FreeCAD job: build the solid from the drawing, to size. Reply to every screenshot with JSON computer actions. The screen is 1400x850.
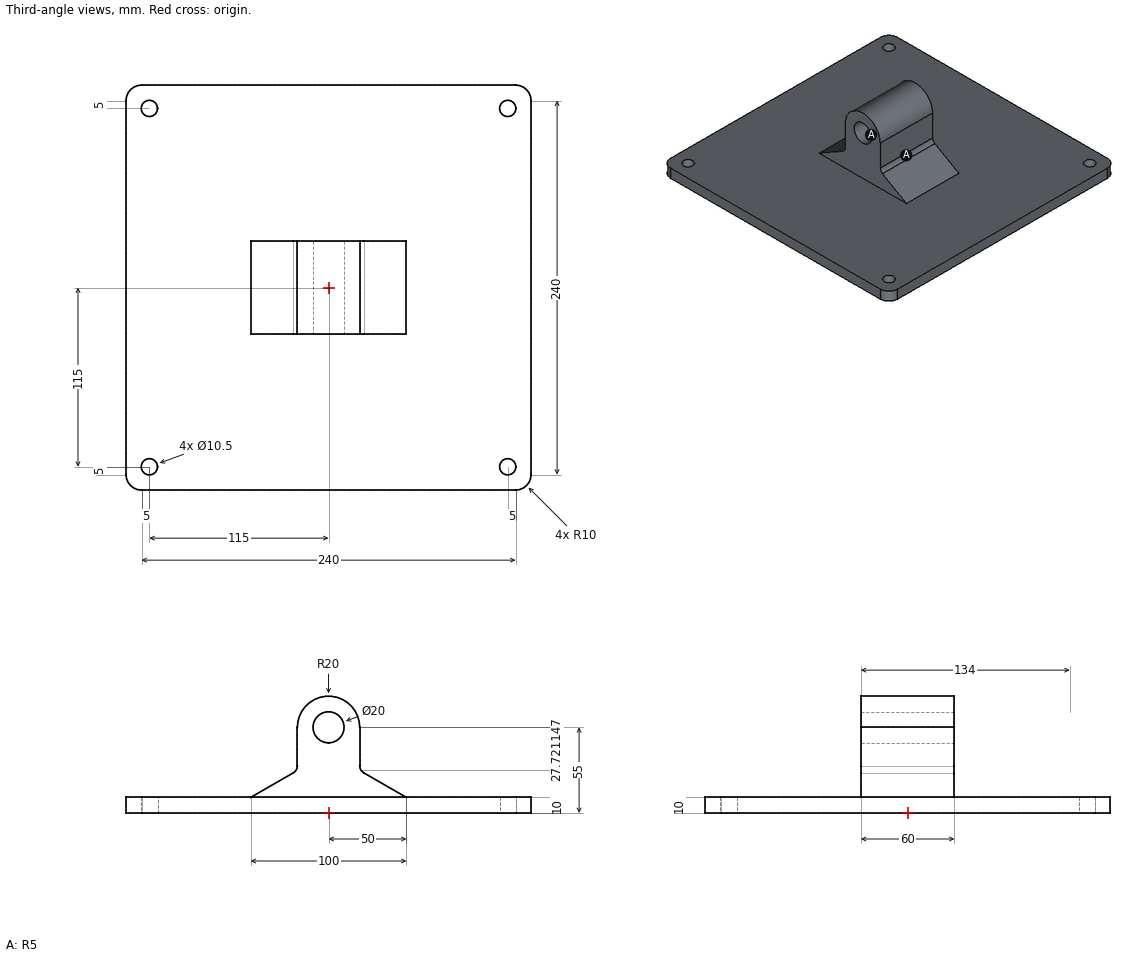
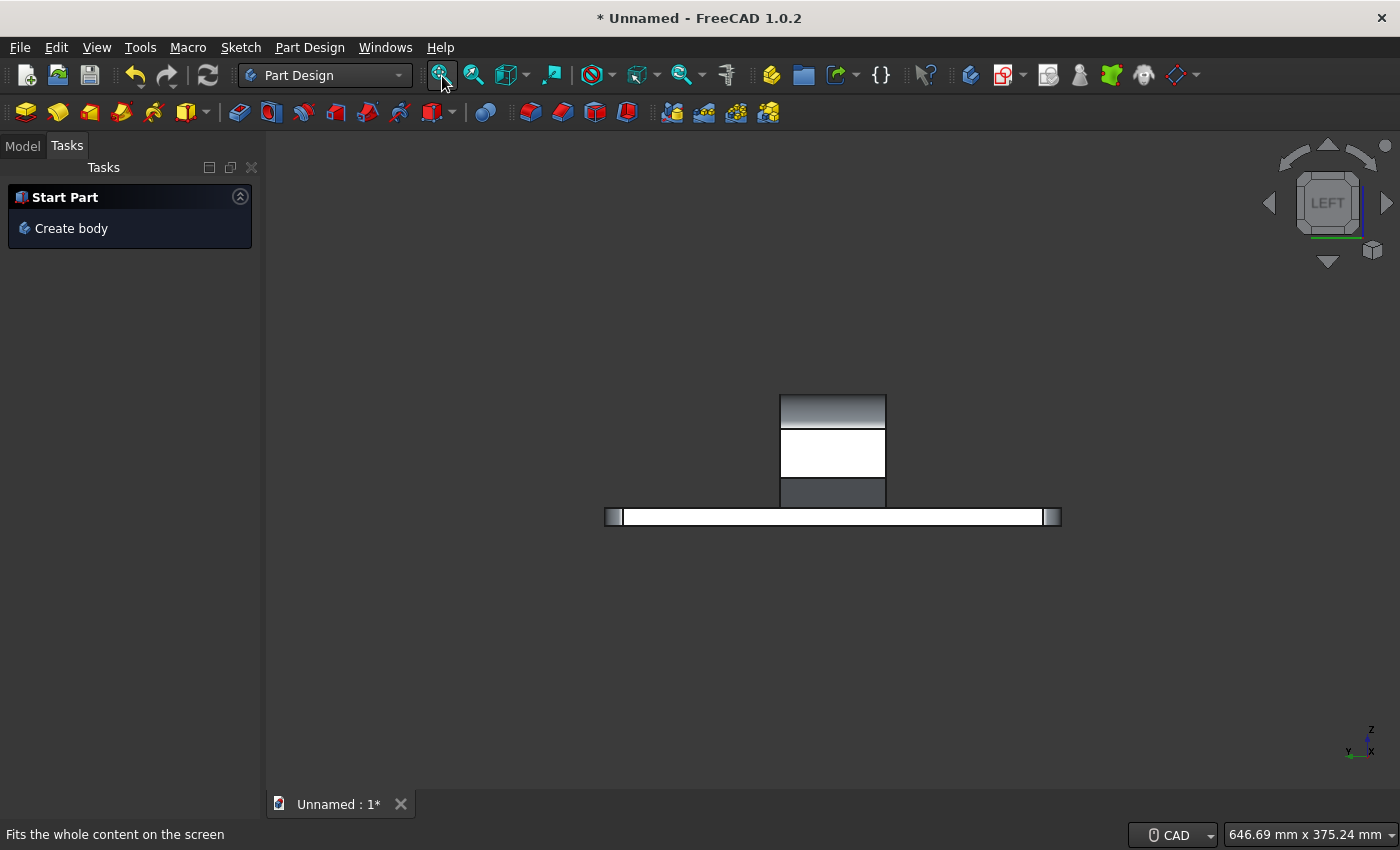
{"action": "left_click", "coordinate": [442, 76]}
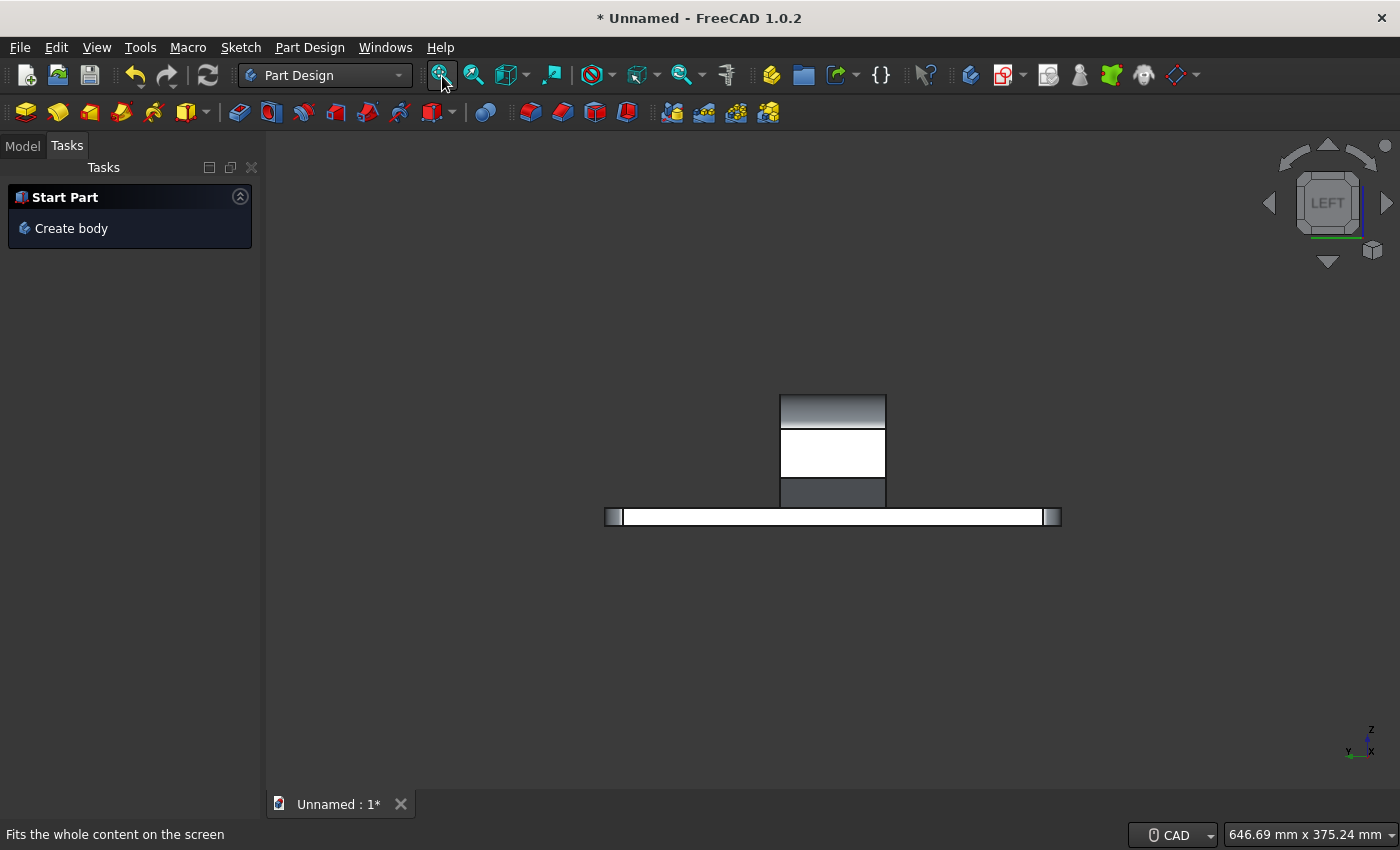
{"action": "key", "text": "v 3"}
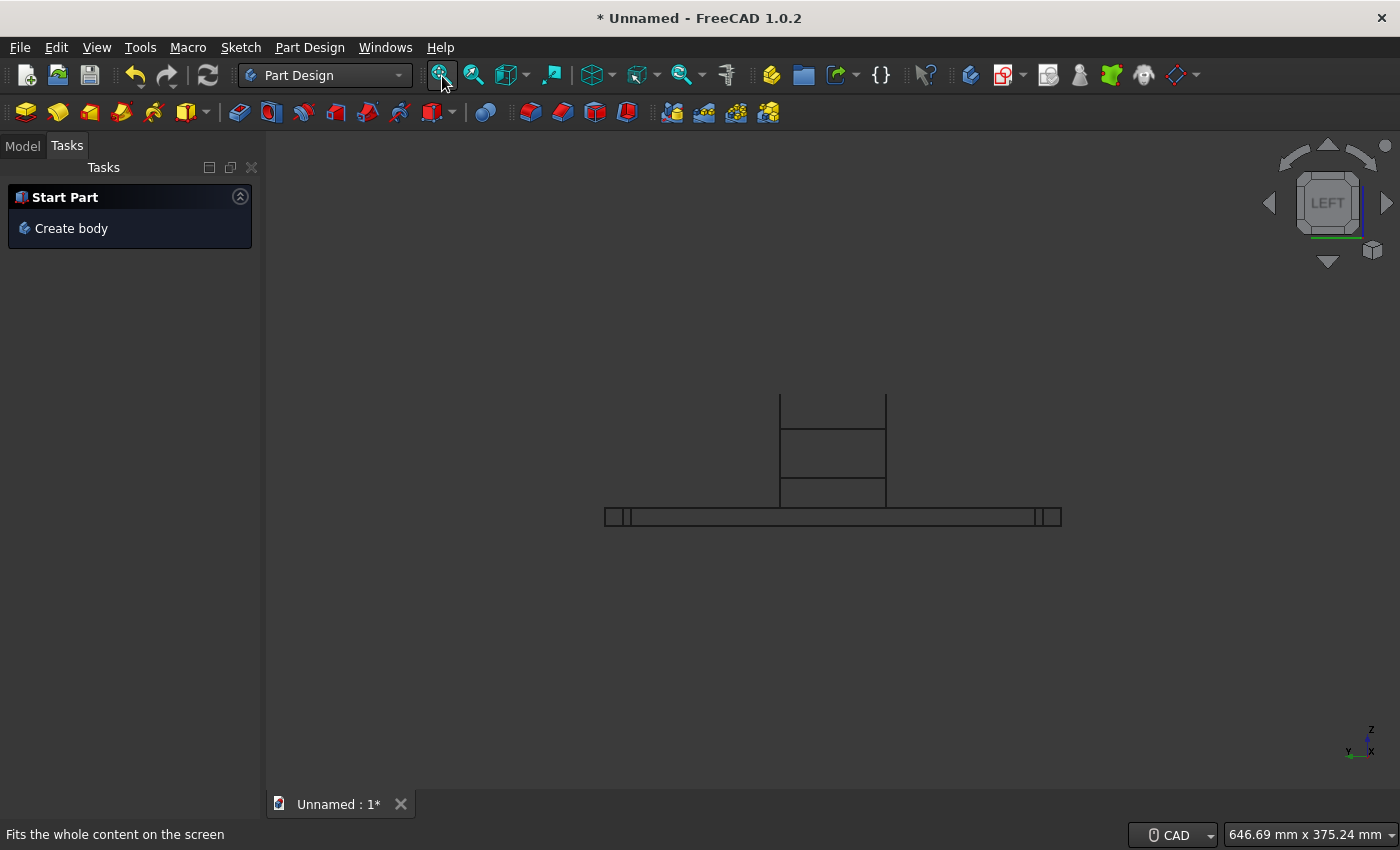
{"action": "key", "text": "0"}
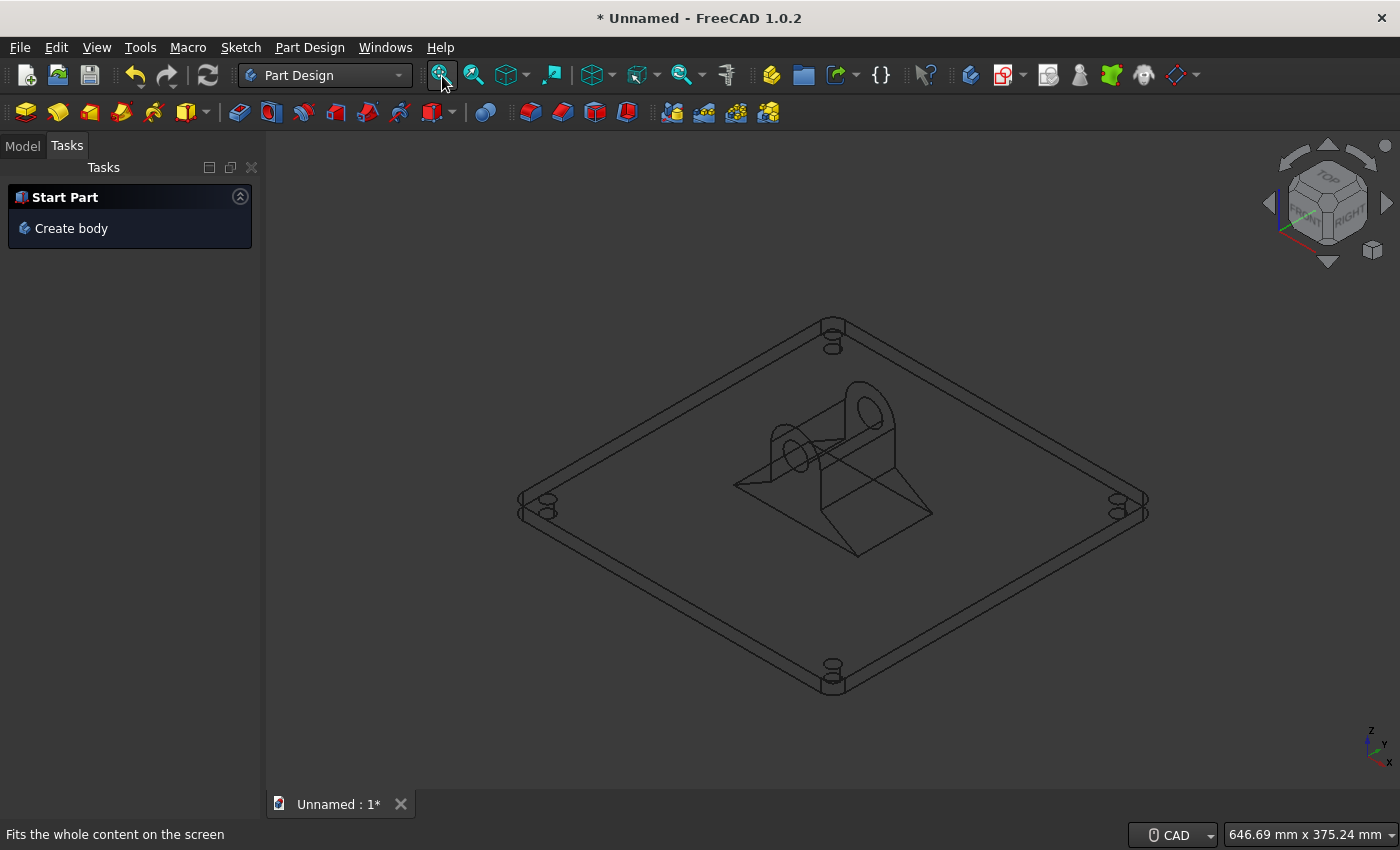
{"action": "left_click", "coordinate": [801, 464]}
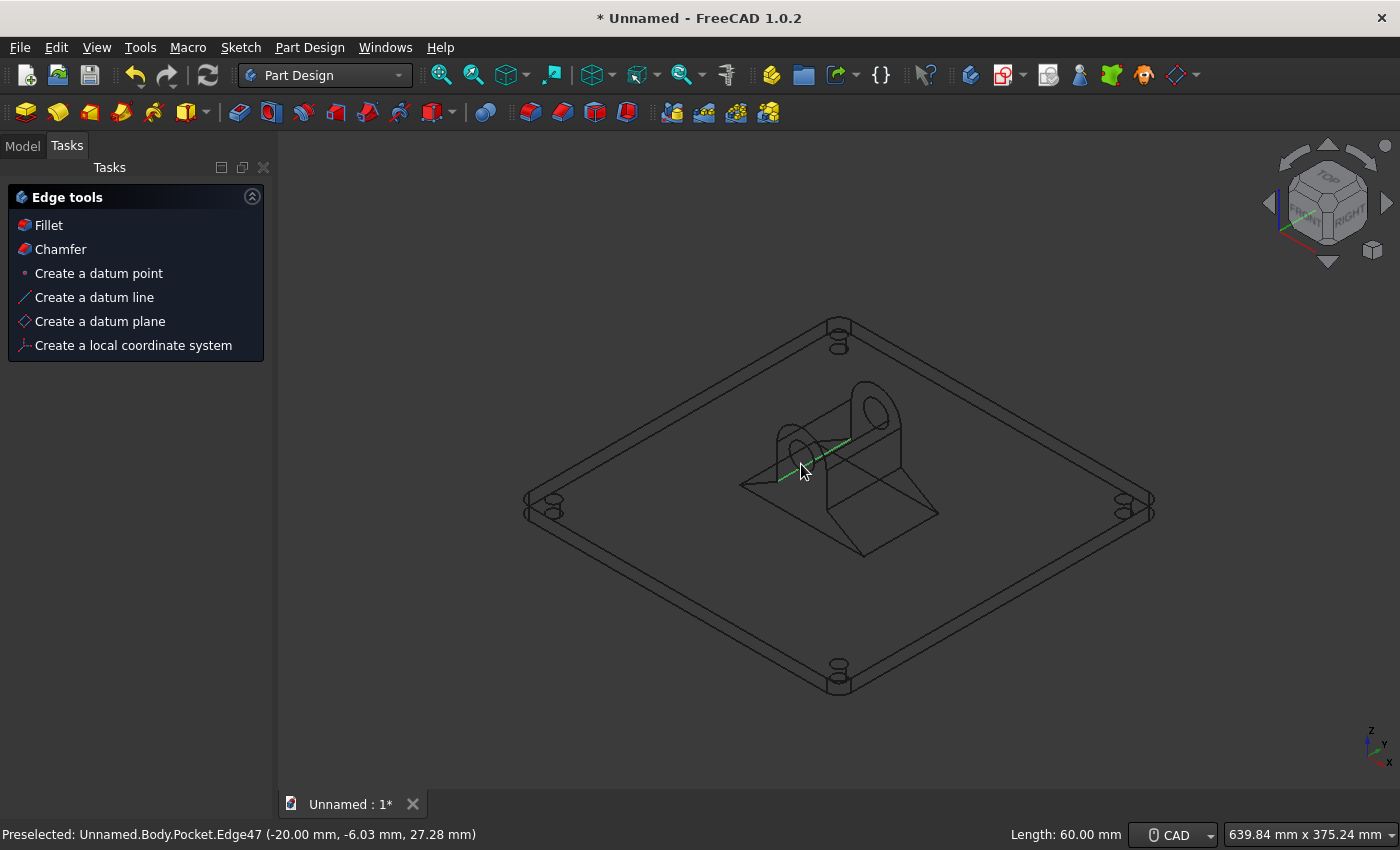
{"action": "left_click", "coordinate": [864, 488], "text": "ctrl"}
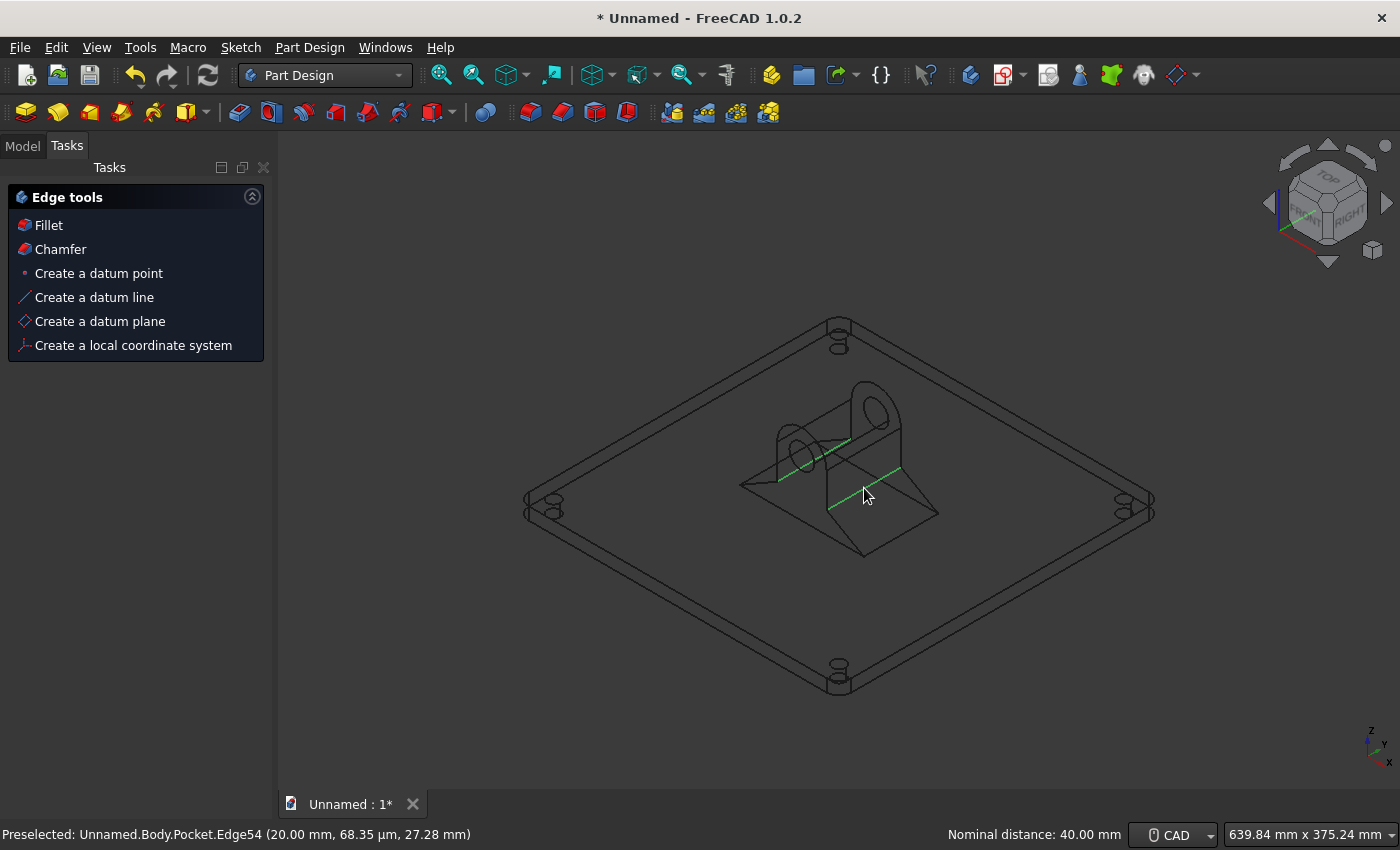
{"action": "key", "text": "v 1"}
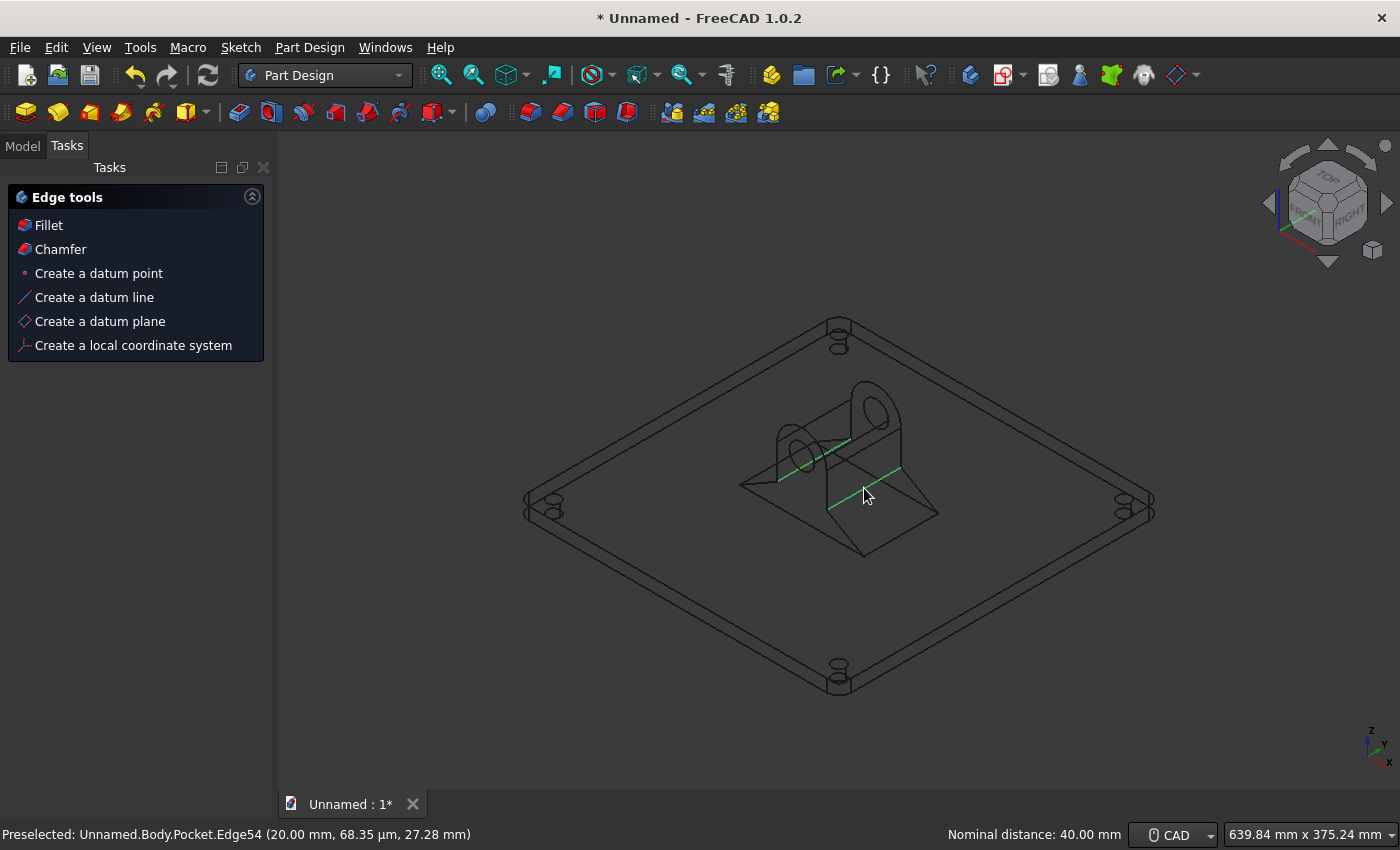
{"action": "left_click", "coordinate": [532, 112]}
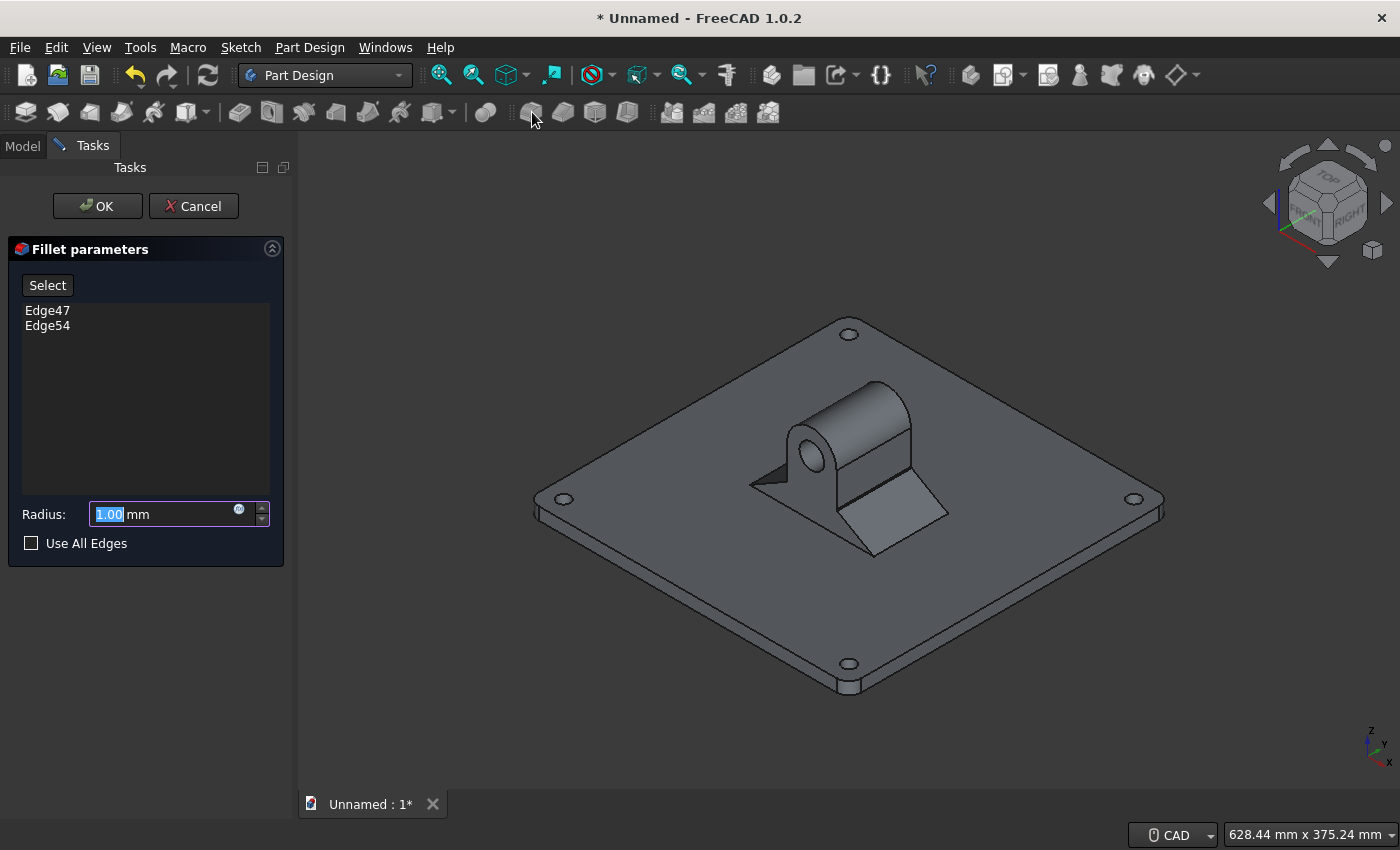
{"action": "type", "text": "5"}
{"action": "key", "text": "Tab"}